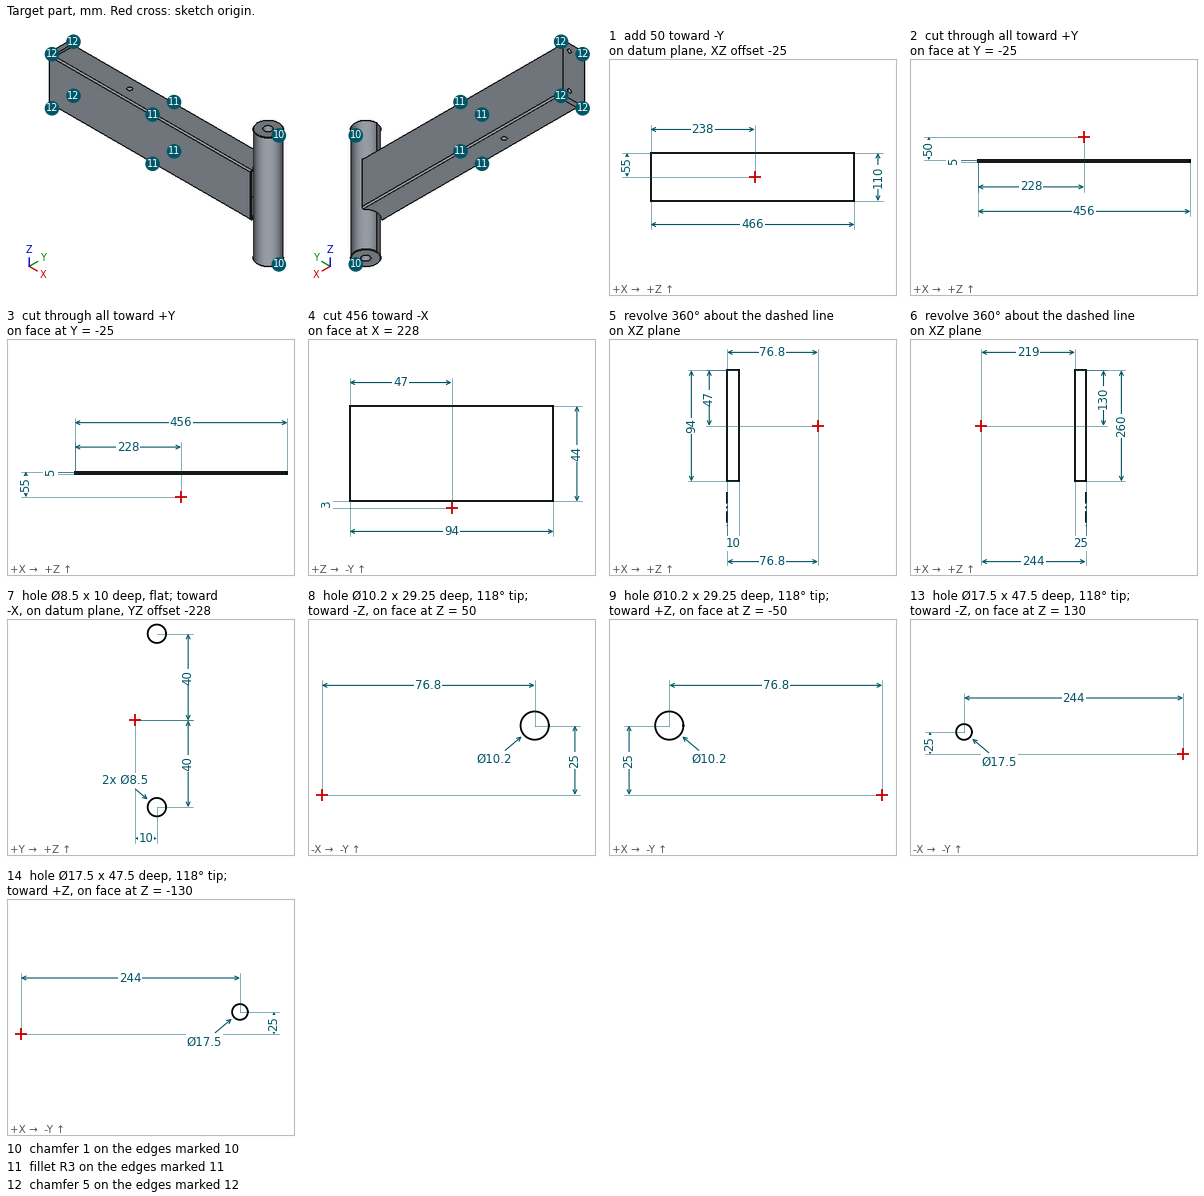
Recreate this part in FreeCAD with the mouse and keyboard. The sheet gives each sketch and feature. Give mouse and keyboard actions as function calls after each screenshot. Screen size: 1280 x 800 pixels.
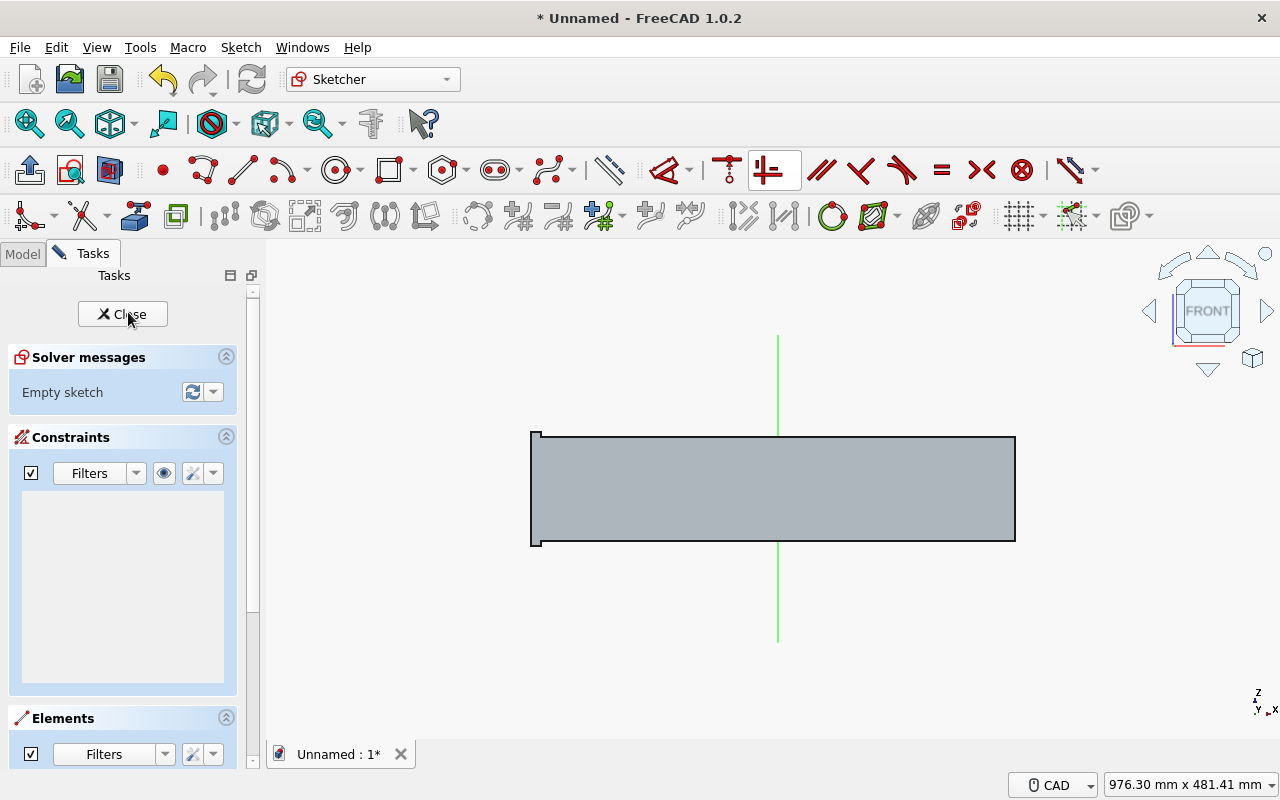
click(110, 170)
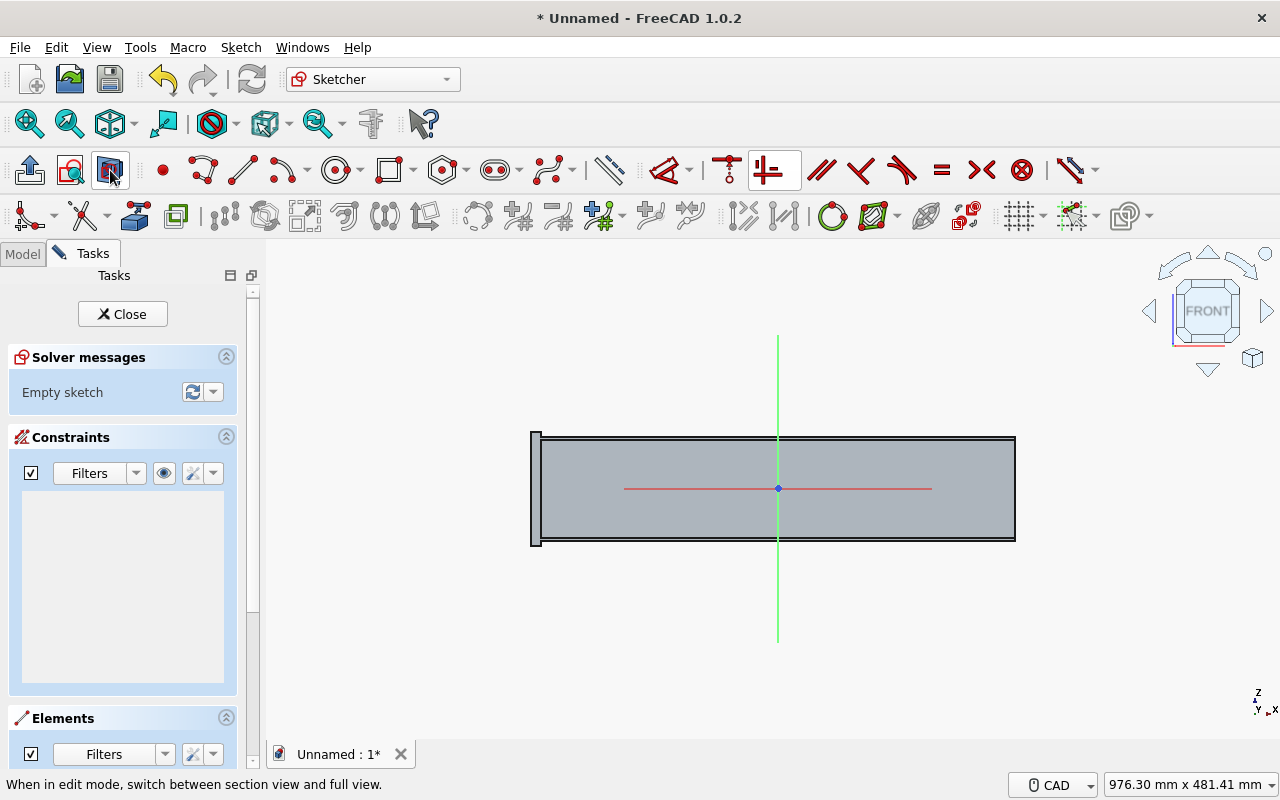
scroll(766, 524, up, 4)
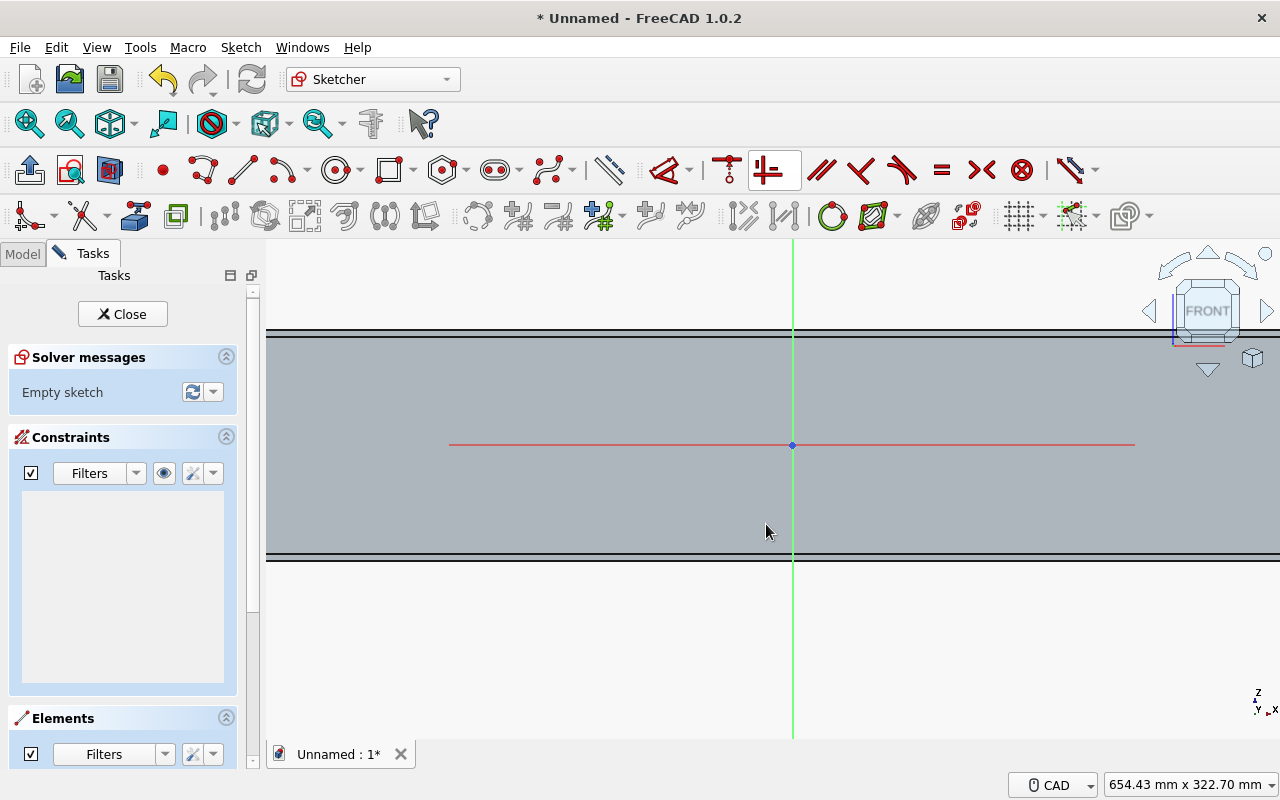
click(390, 170)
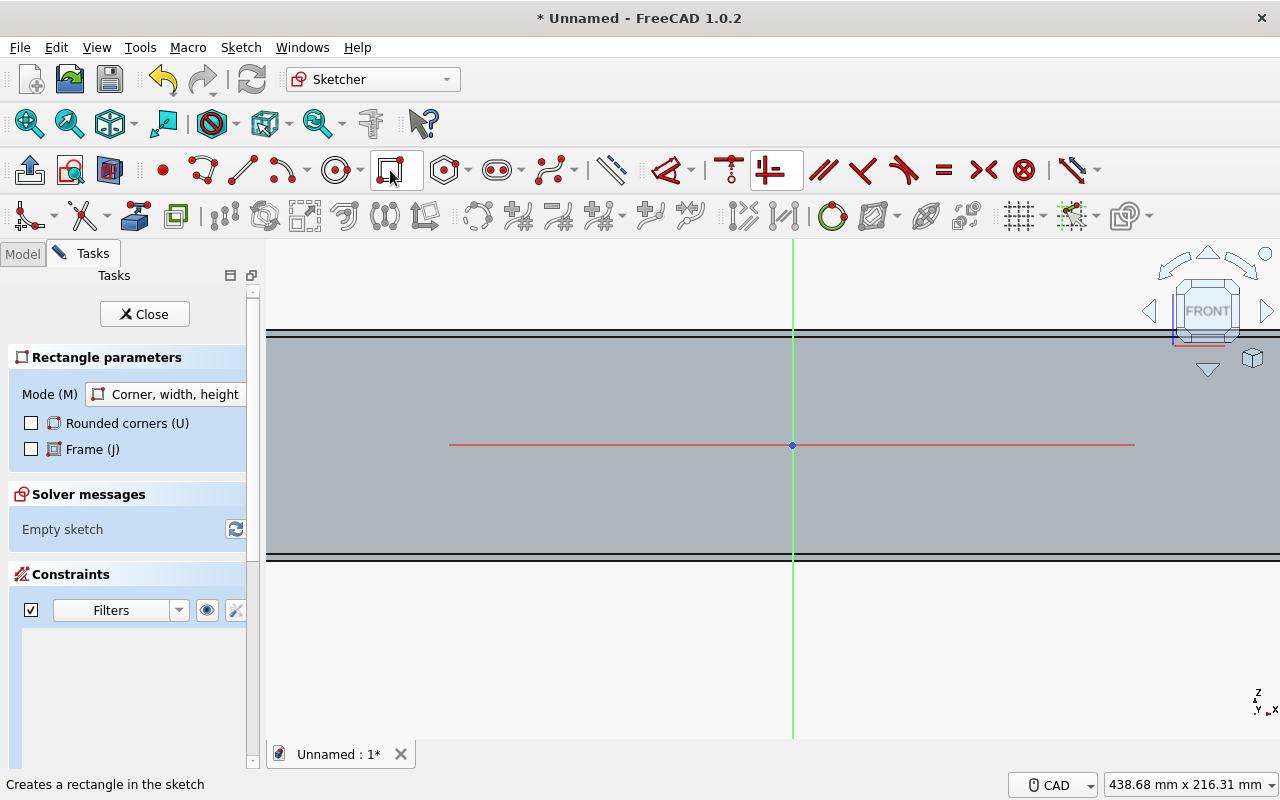
click(615, 337)
move(638, 554)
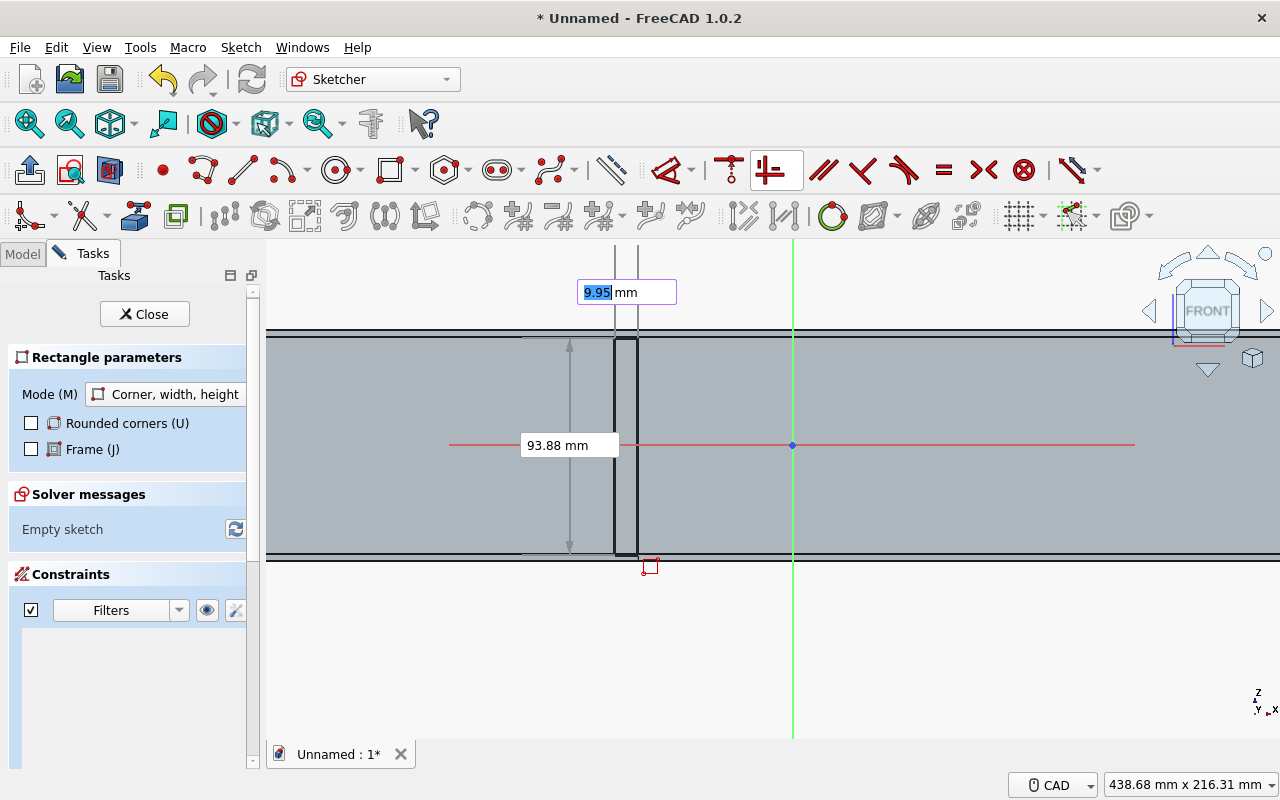
text(10)
key(Tab)
text(94)
key(Return)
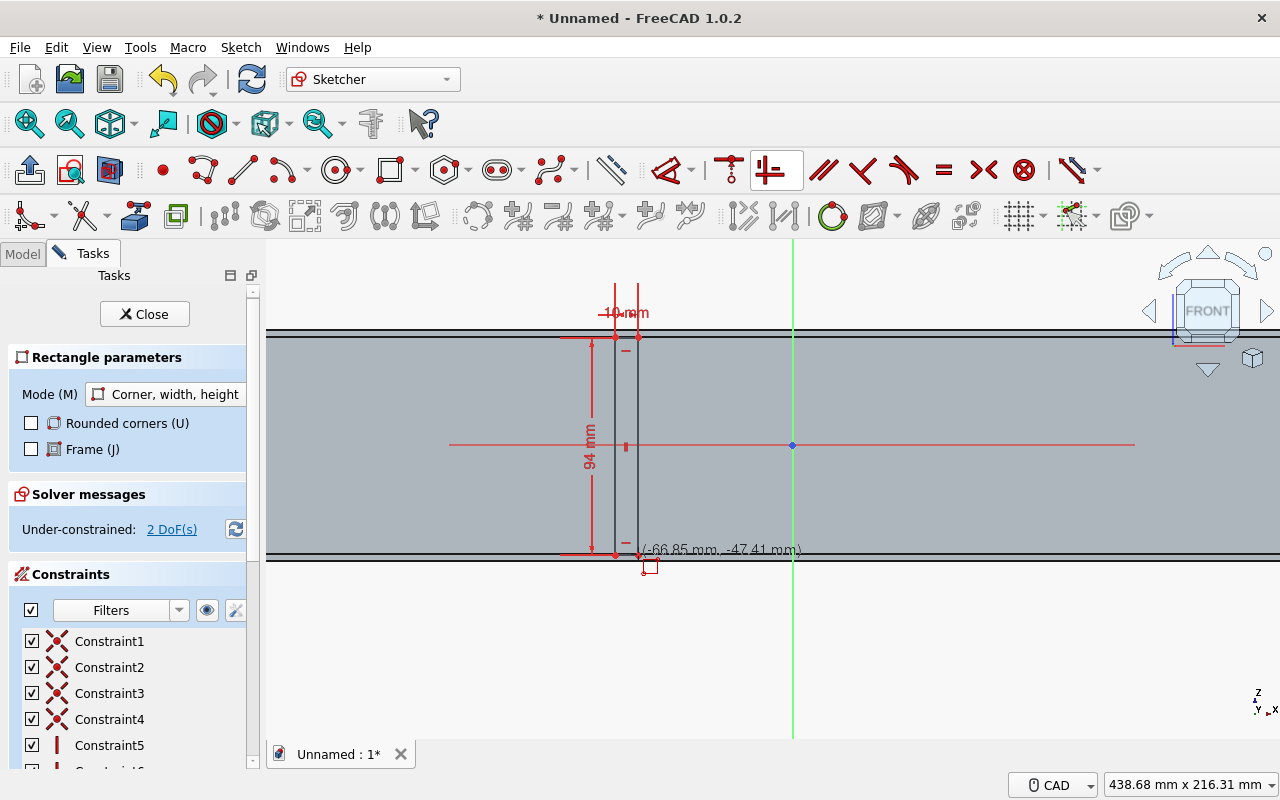
click(244, 170)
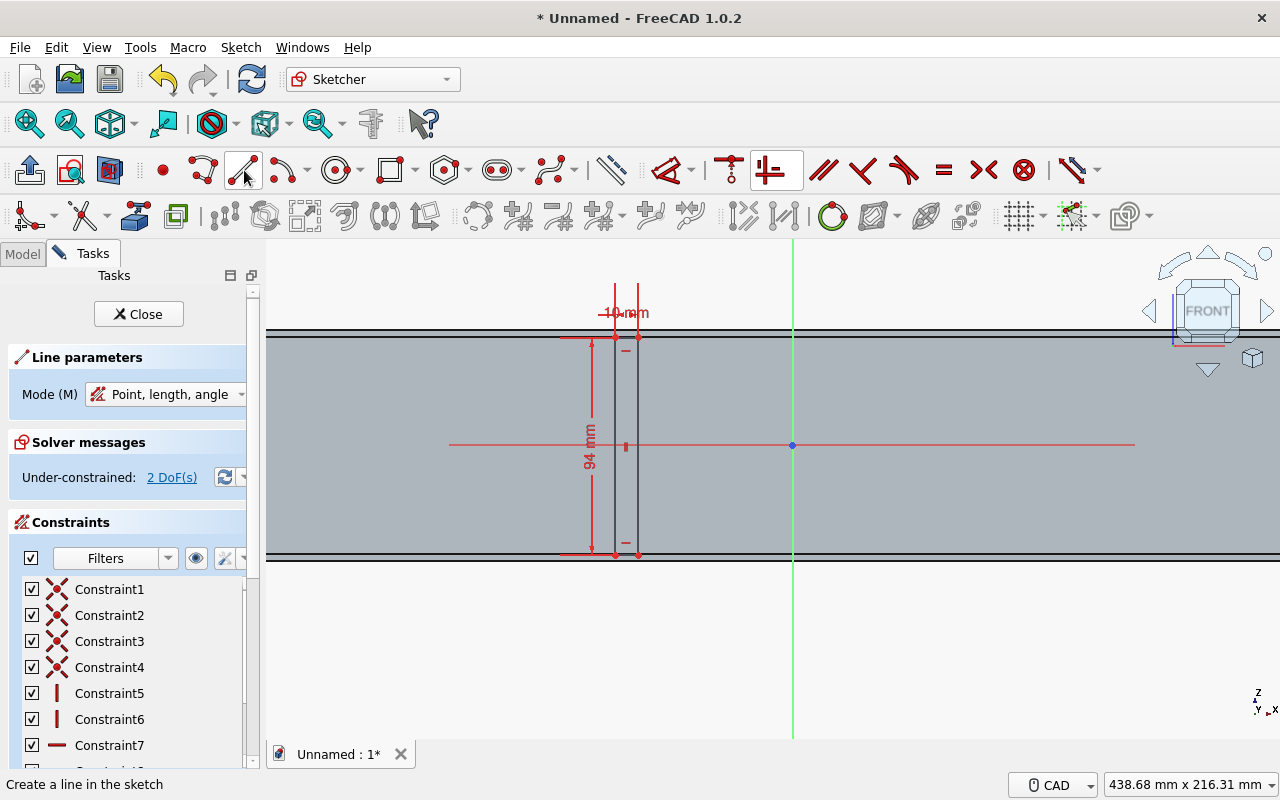
click(615, 576)
click(615, 641)
key(Escape)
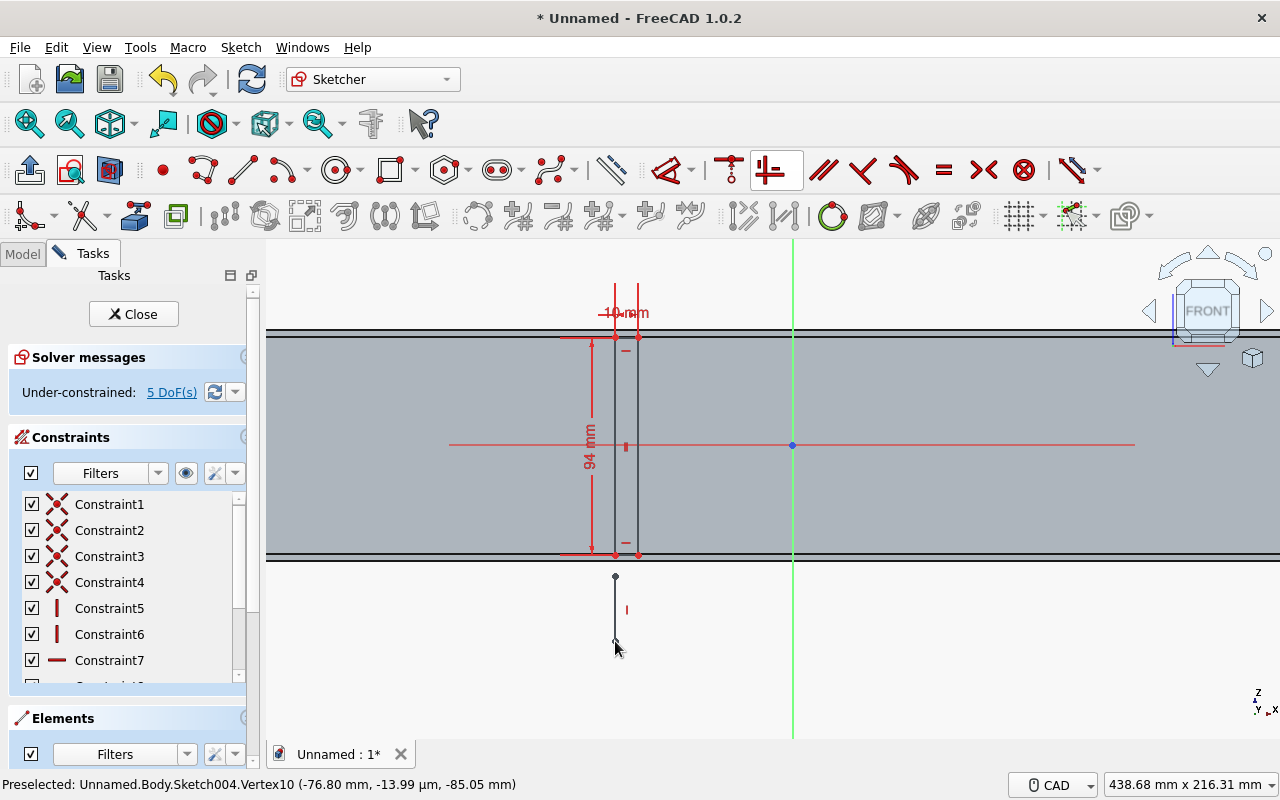
click(615, 596)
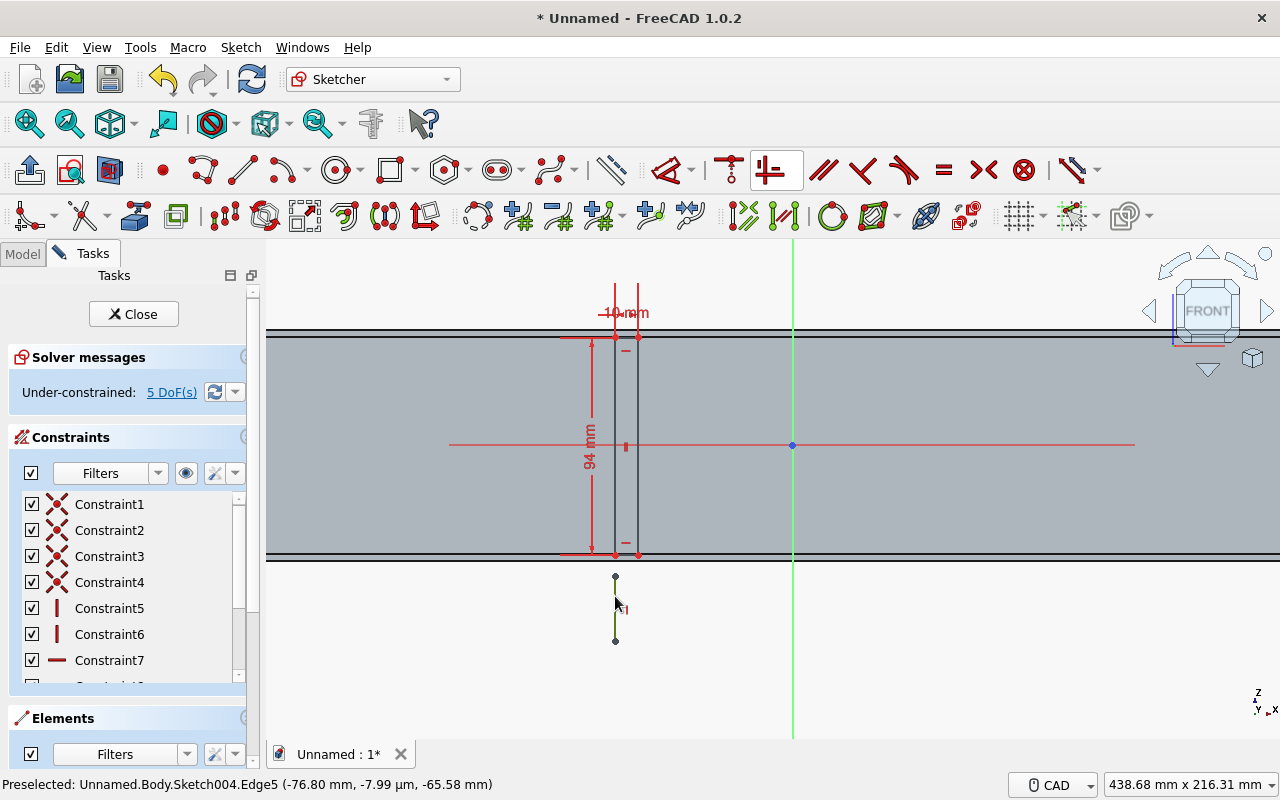
click(612, 170)